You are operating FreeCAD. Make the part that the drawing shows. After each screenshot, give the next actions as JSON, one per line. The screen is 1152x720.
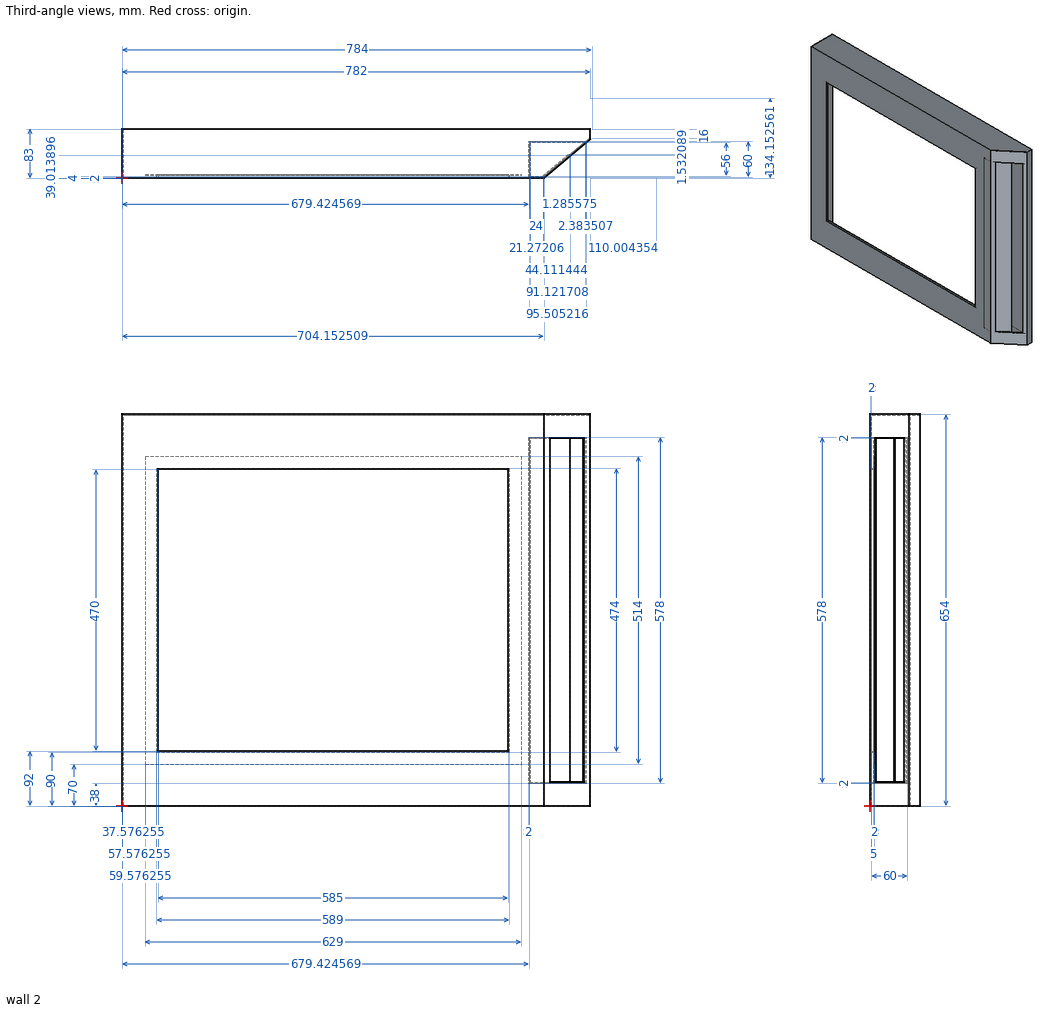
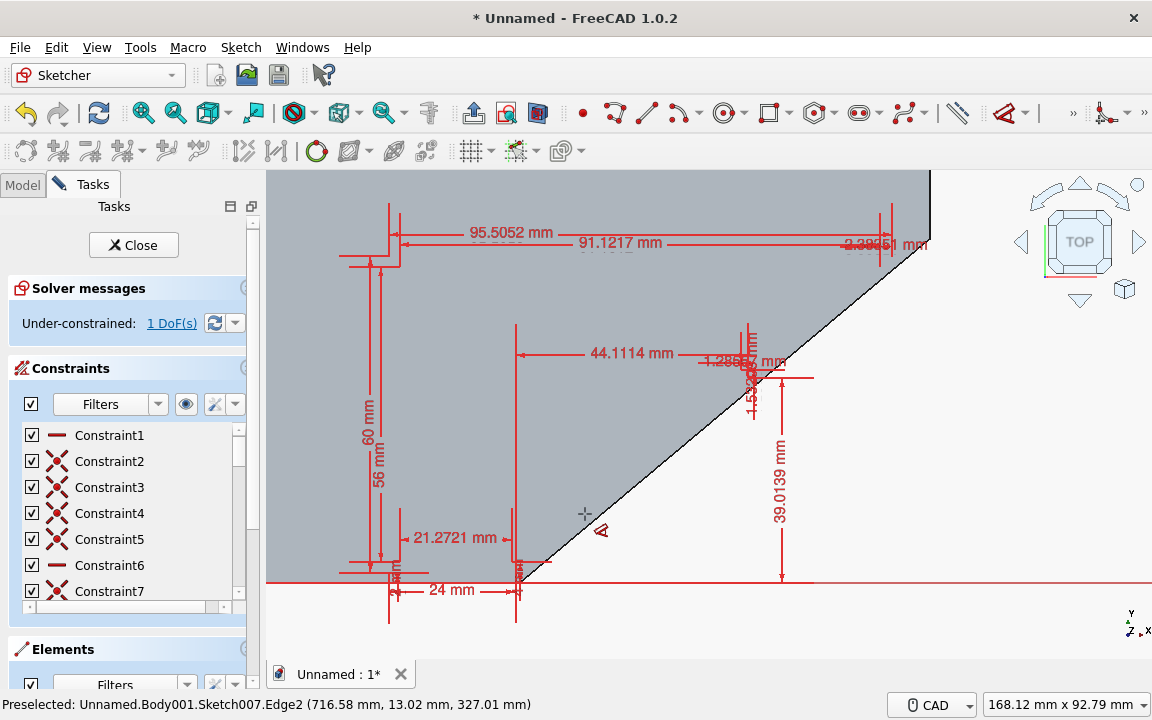
{"action": "left_click", "coordinate": [389, 573]}
{"action": "left_click", "coordinate": [342, 617]}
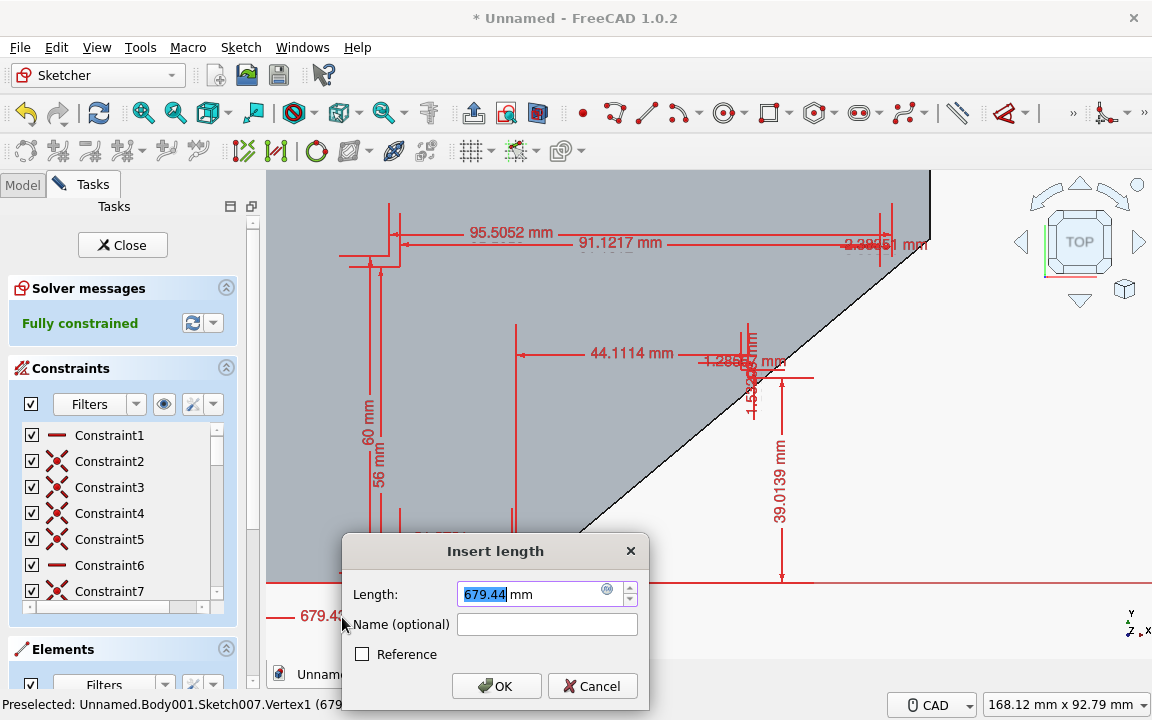
{"action": "type", "text": "679.424569"}
{"action": "key", "text": "Return"}
{"action": "key", "text": "Escape"}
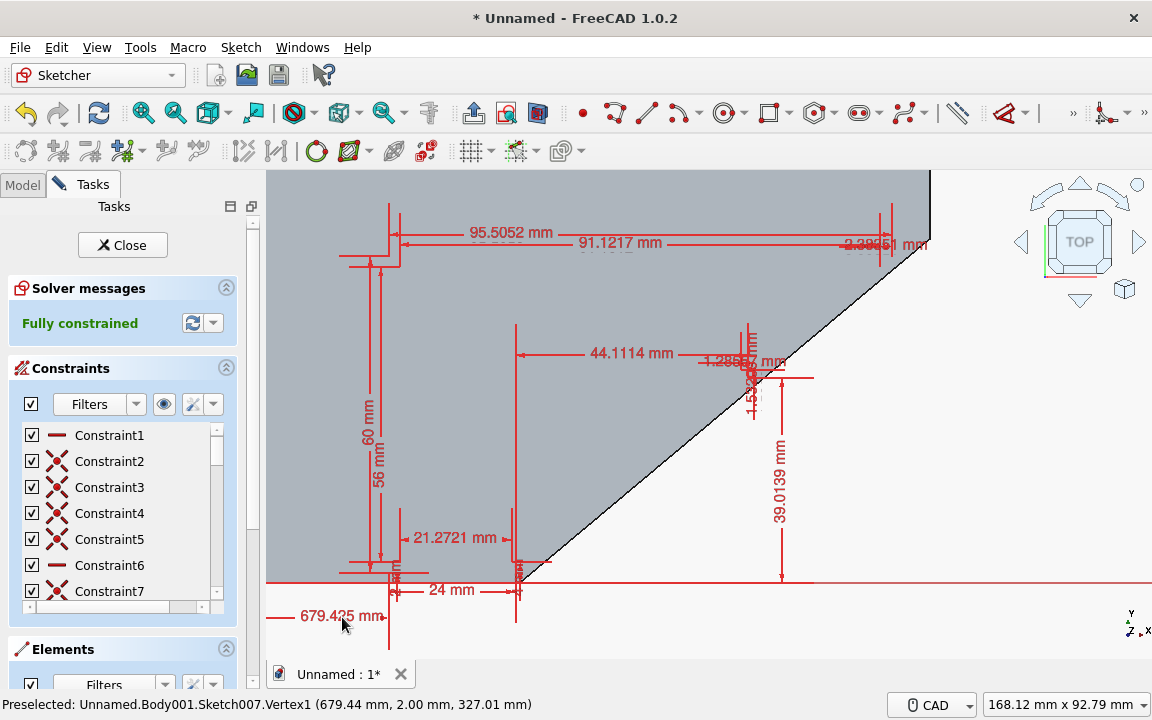
{"action": "left_click", "coordinate": [123, 245]}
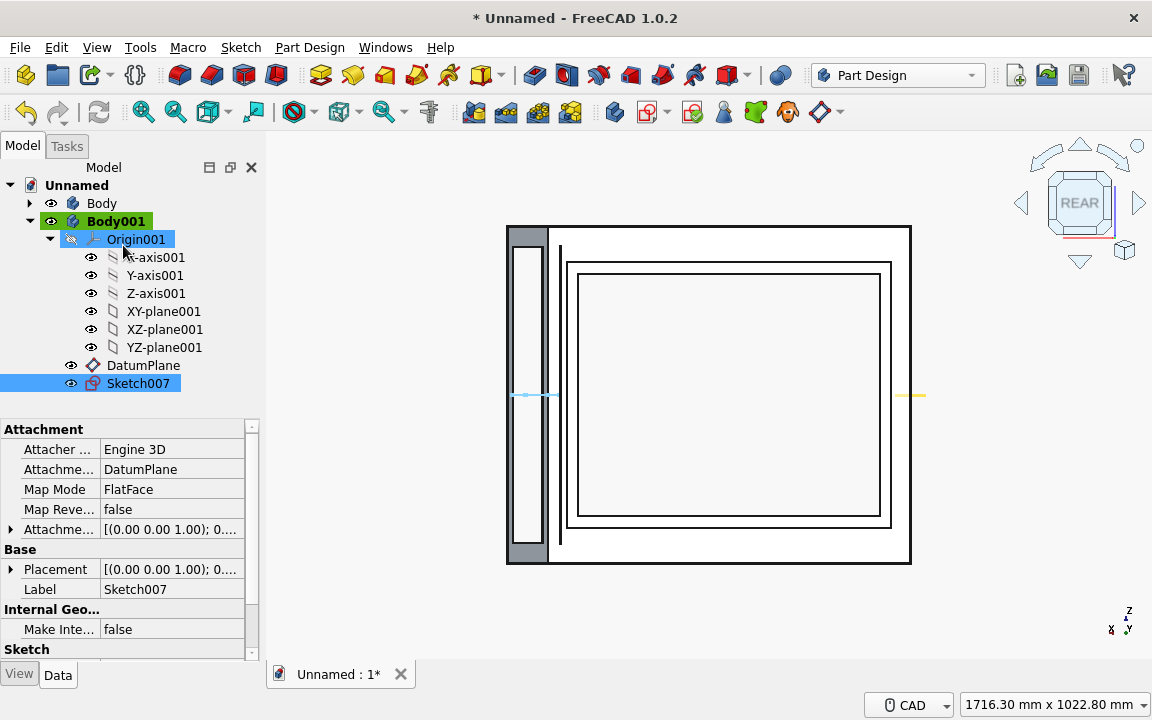
{"action": "left_click", "coordinate": [322, 76]}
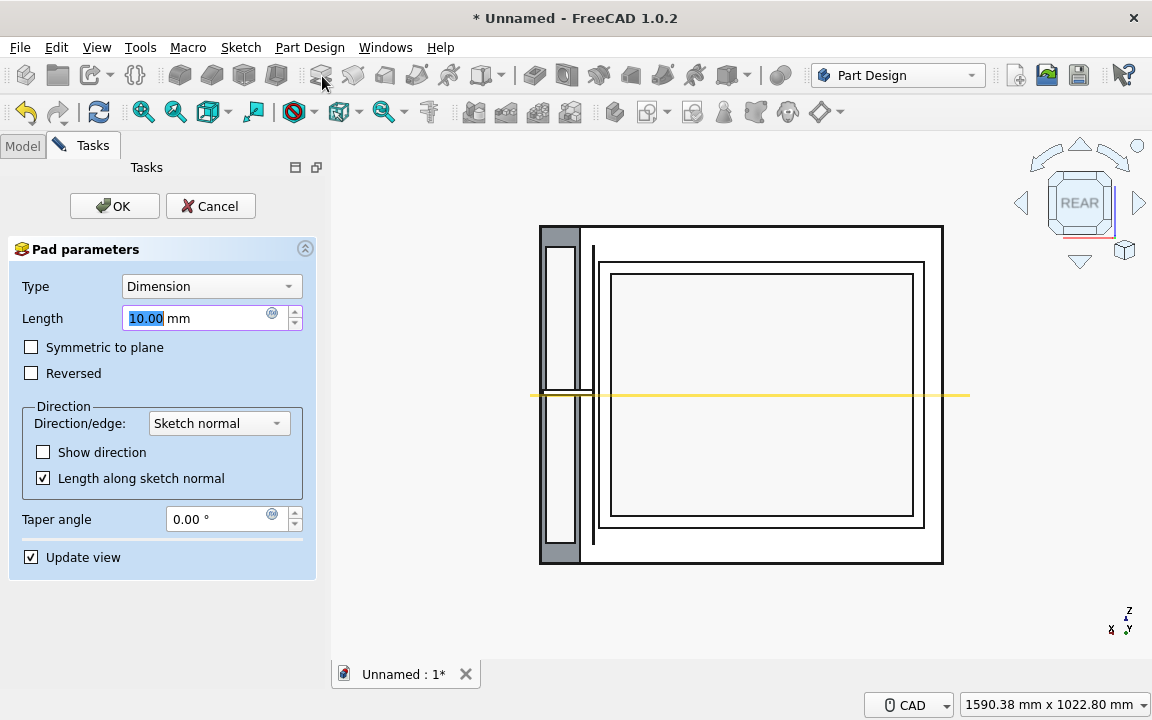
{"action": "type", "text": "578"}
{"action": "key", "text": "Tab"}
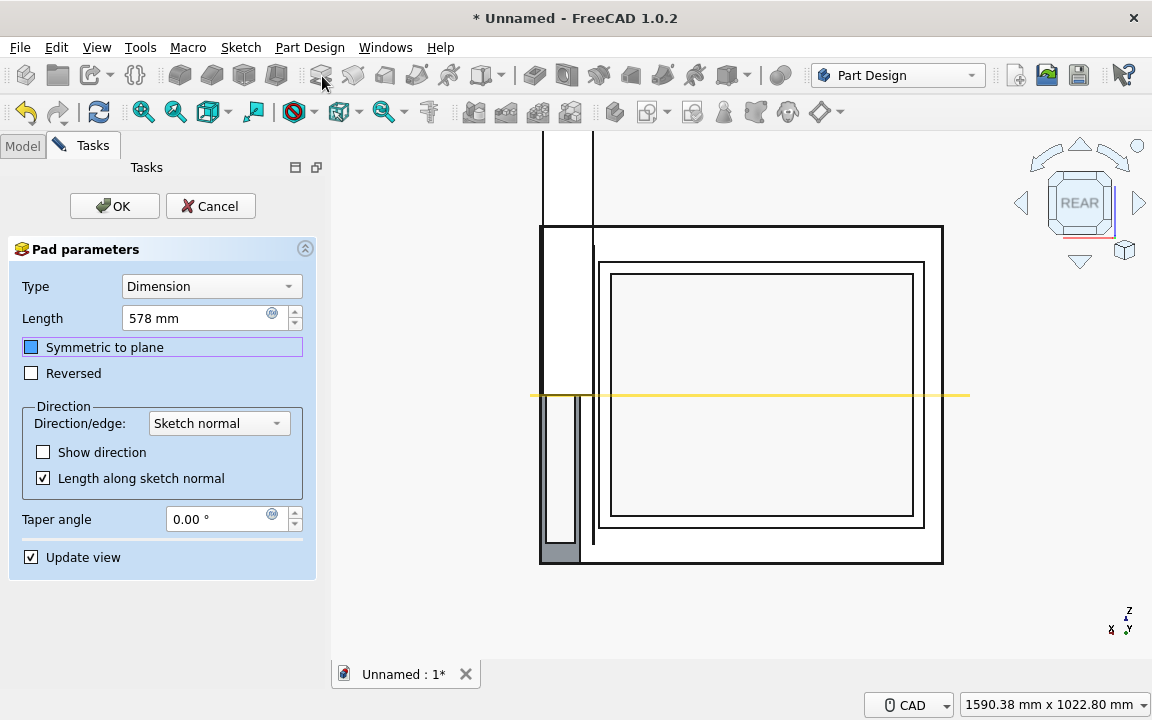
{"action": "left_click", "coordinate": [30, 347]}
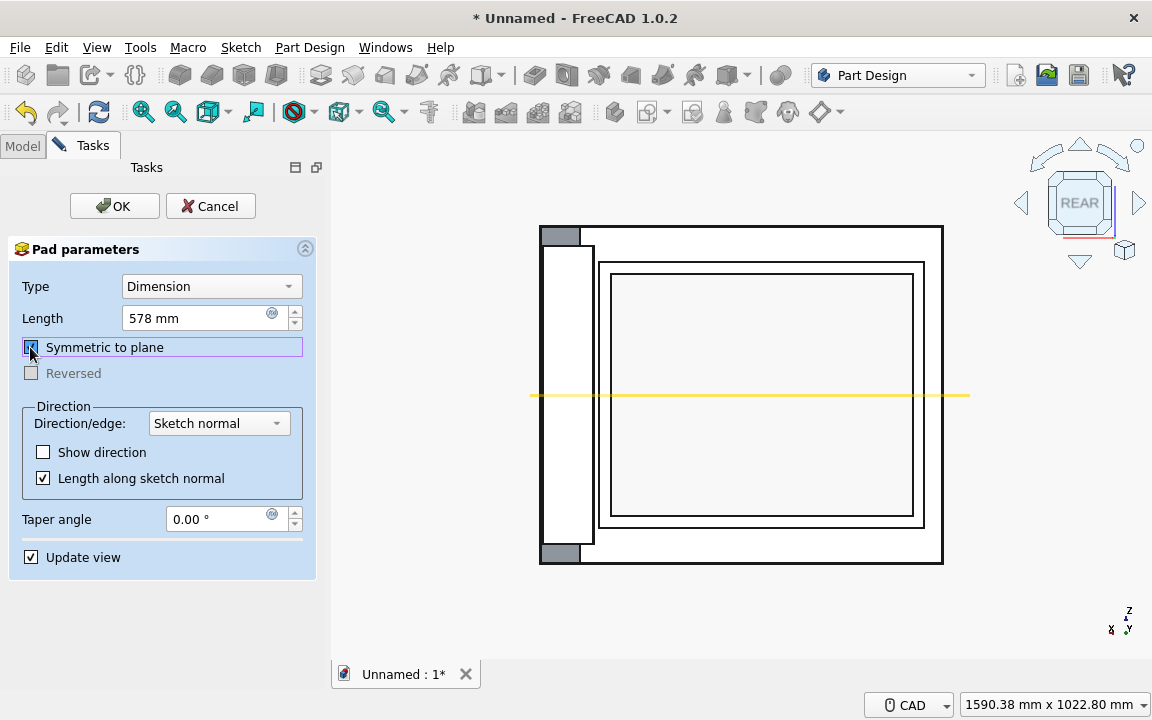
{"action": "left_click", "coordinate": [115, 206]}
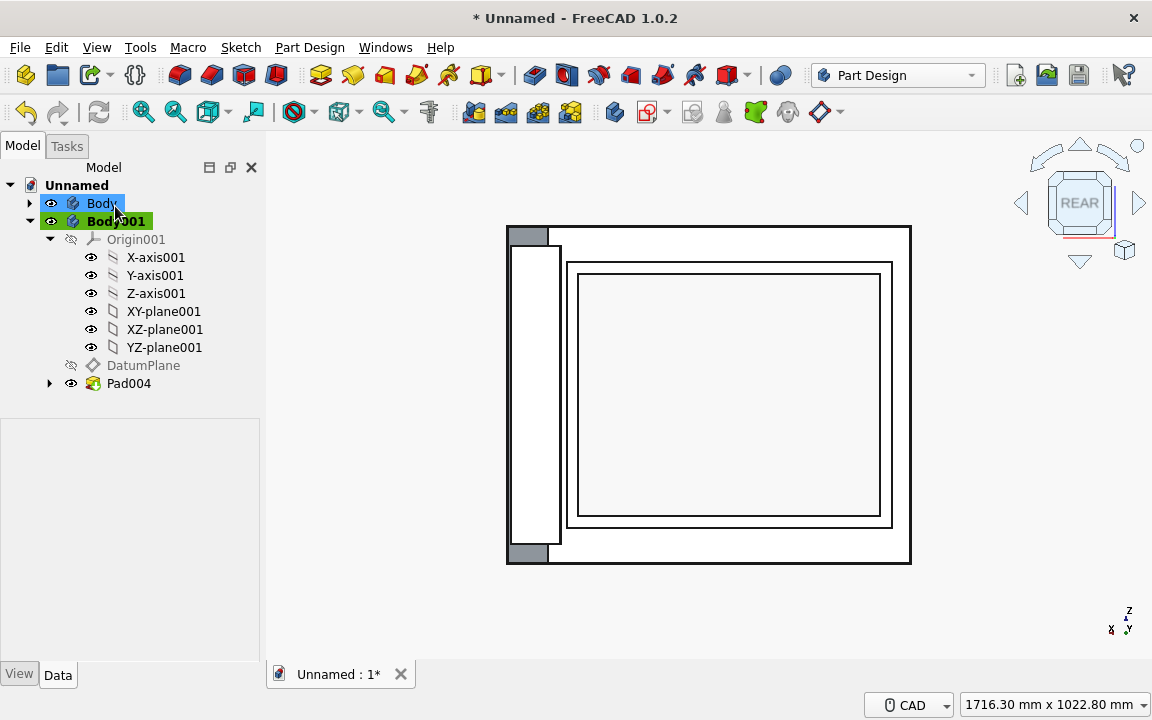
{"action": "left_click", "coordinate": [616, 112]}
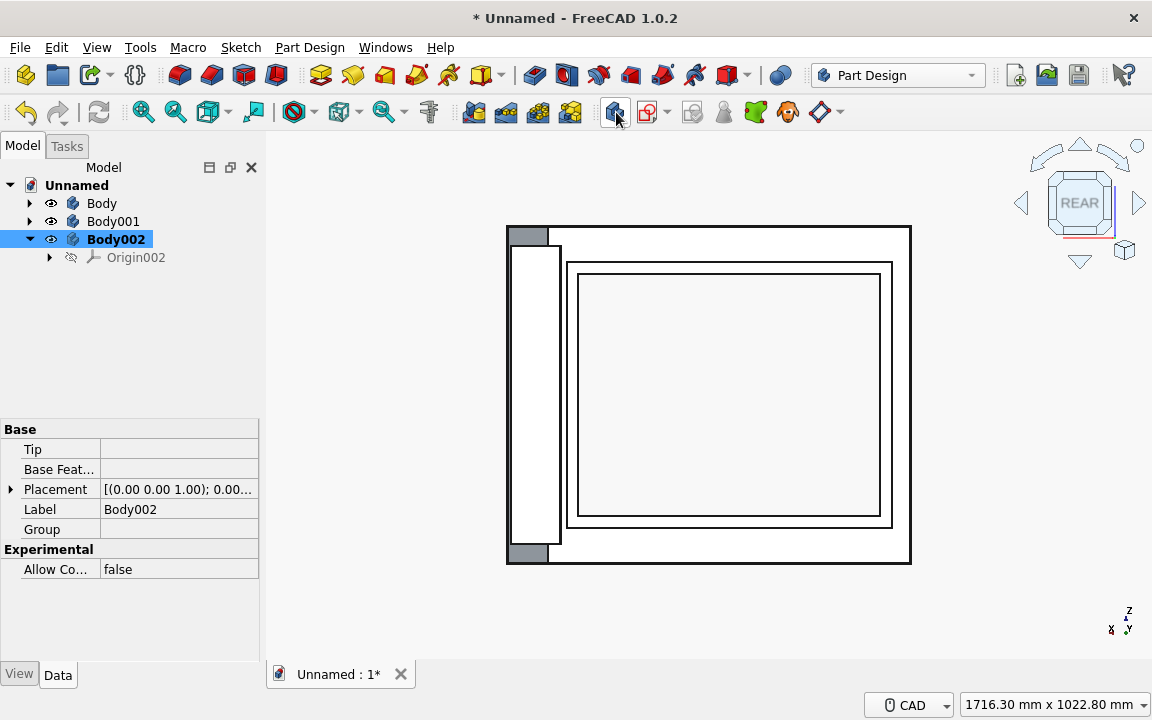
{"action": "left_click", "coordinate": [50, 257]}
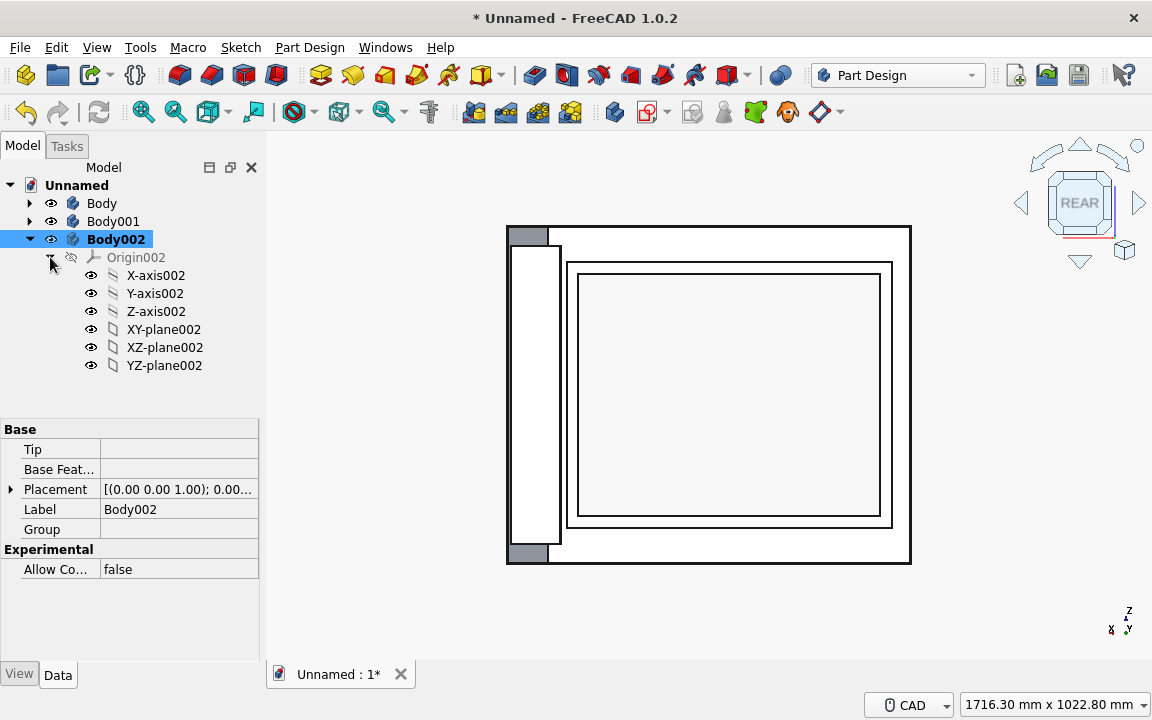
{"action": "left_click", "coordinate": [136, 329]}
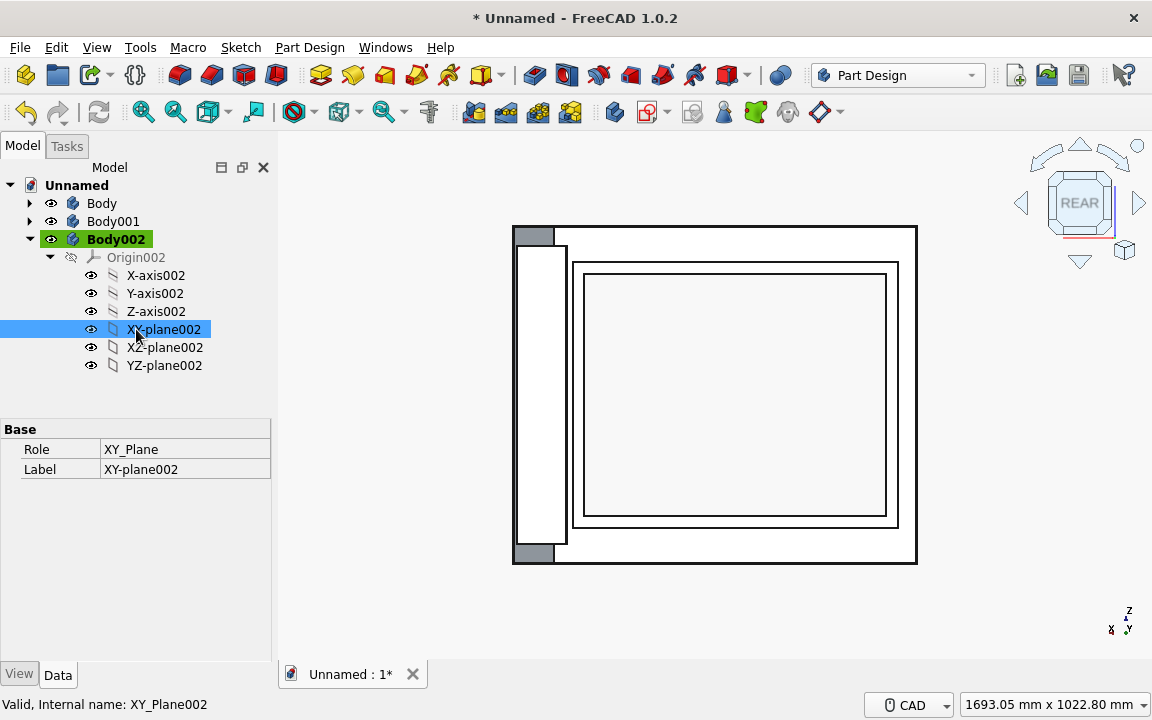
{"action": "left_click", "coordinate": [820, 112]}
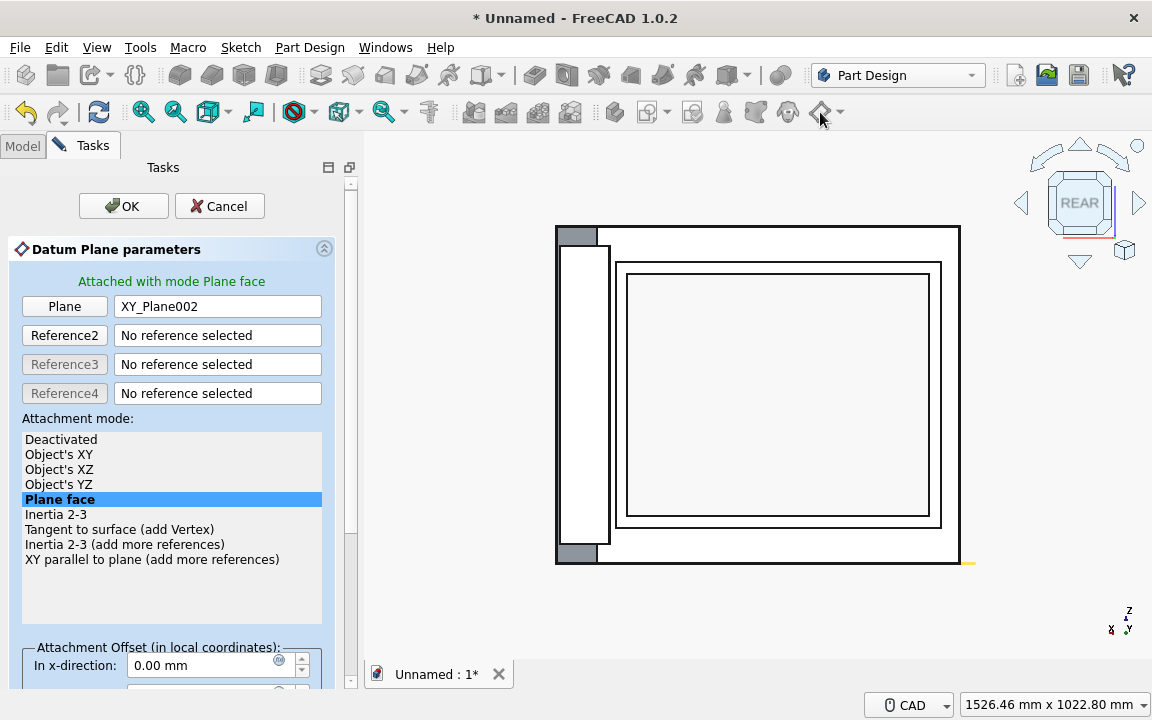
{"action": "scroll", "coordinate": [351, 432], "scroll_direction": "down", "scroll_amount": 2}